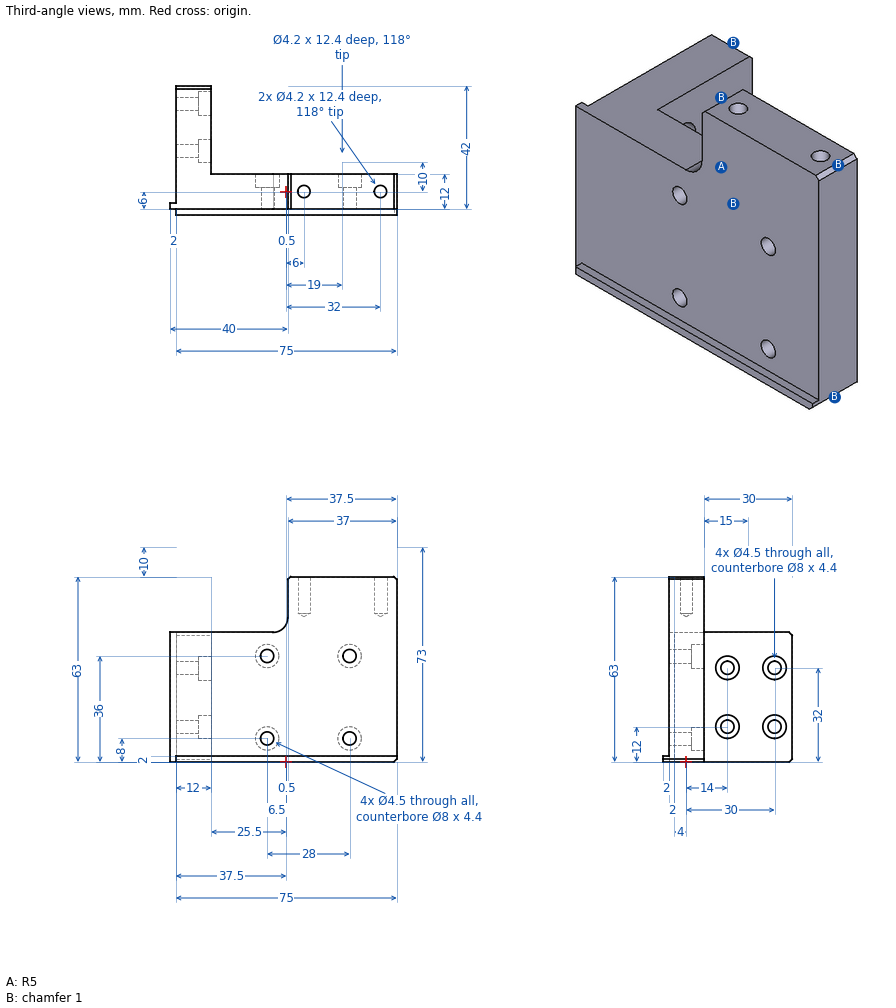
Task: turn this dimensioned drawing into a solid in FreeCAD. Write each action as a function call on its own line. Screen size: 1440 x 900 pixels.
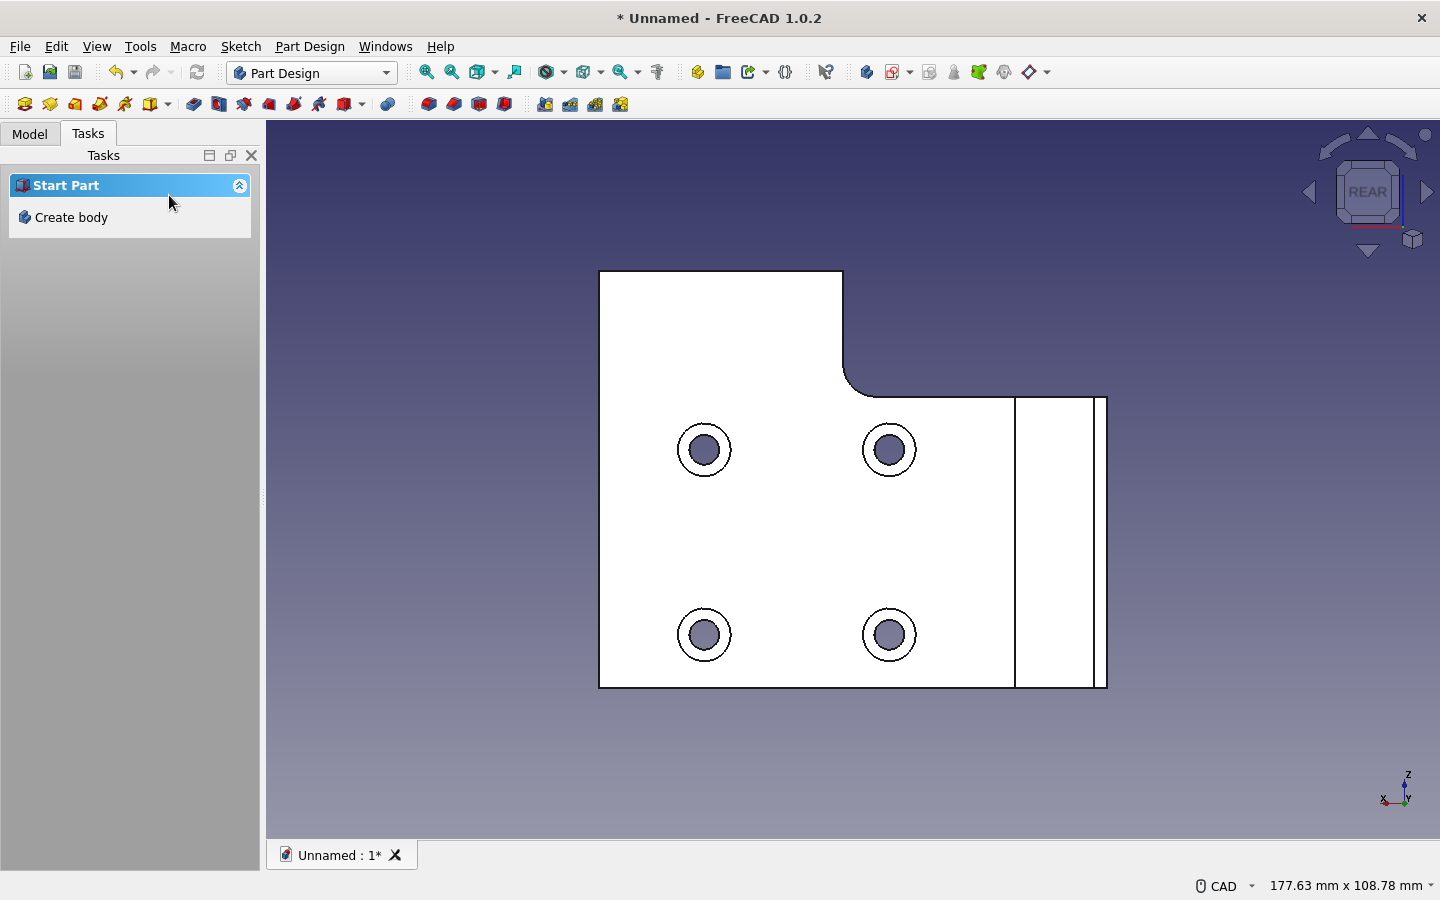
click(1055, 687)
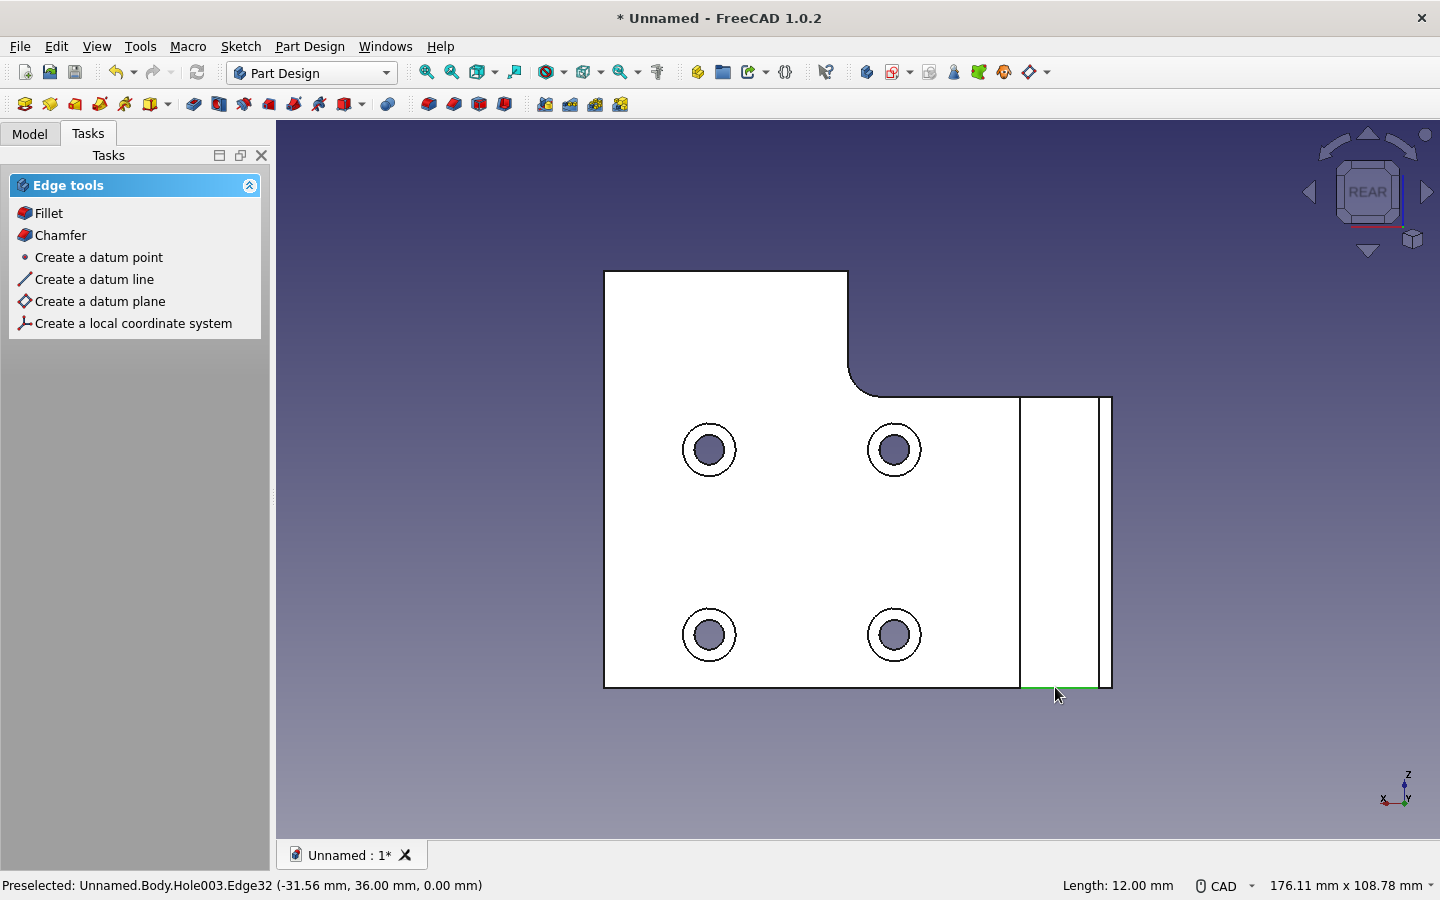
click(1060, 396, ctrl)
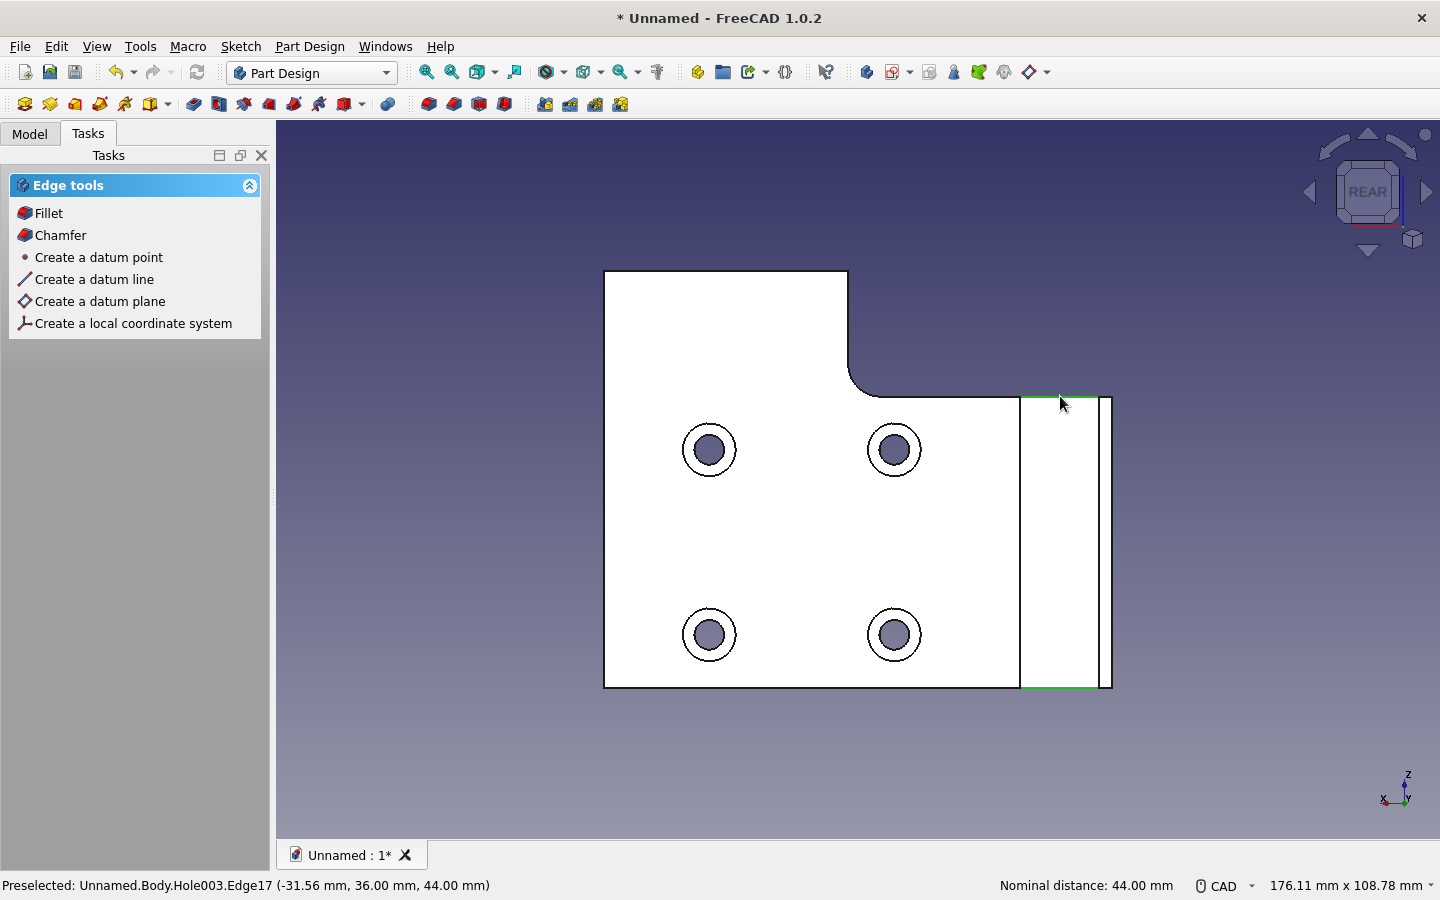
key(0)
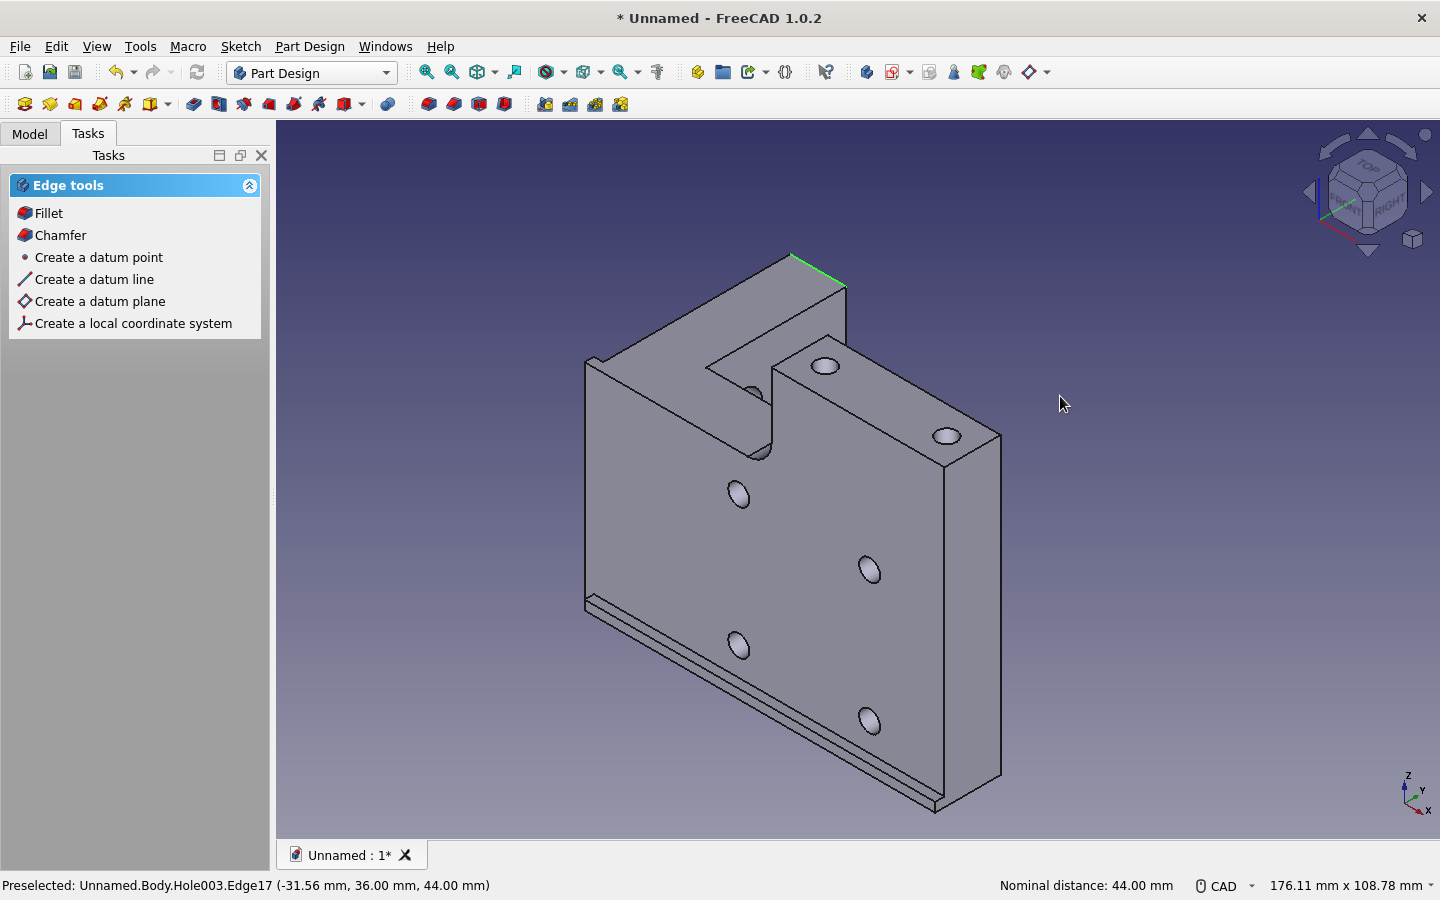
click(973, 450, ctrl)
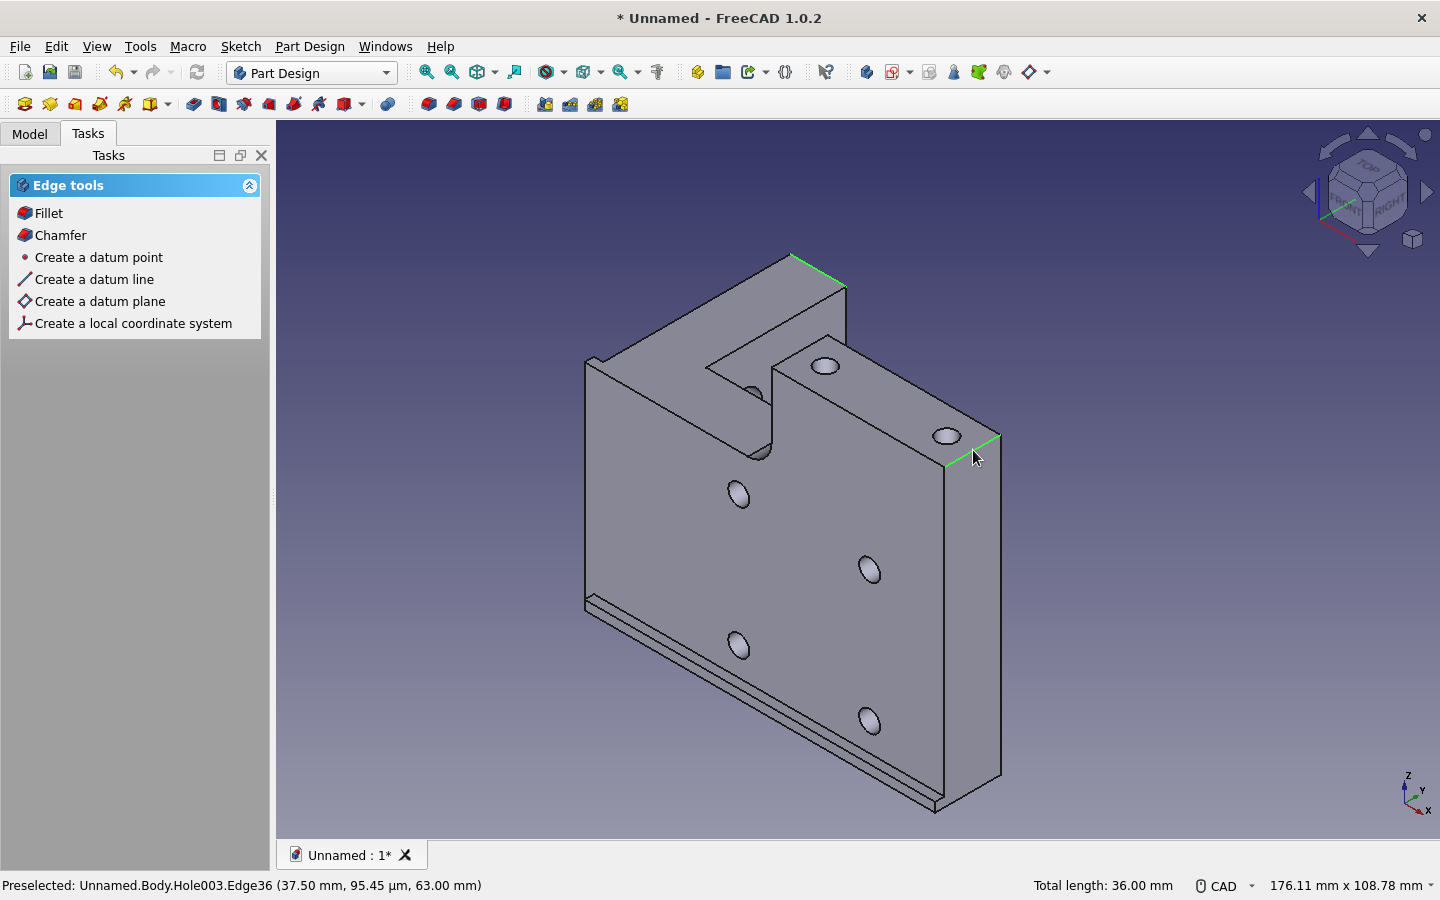
key(2)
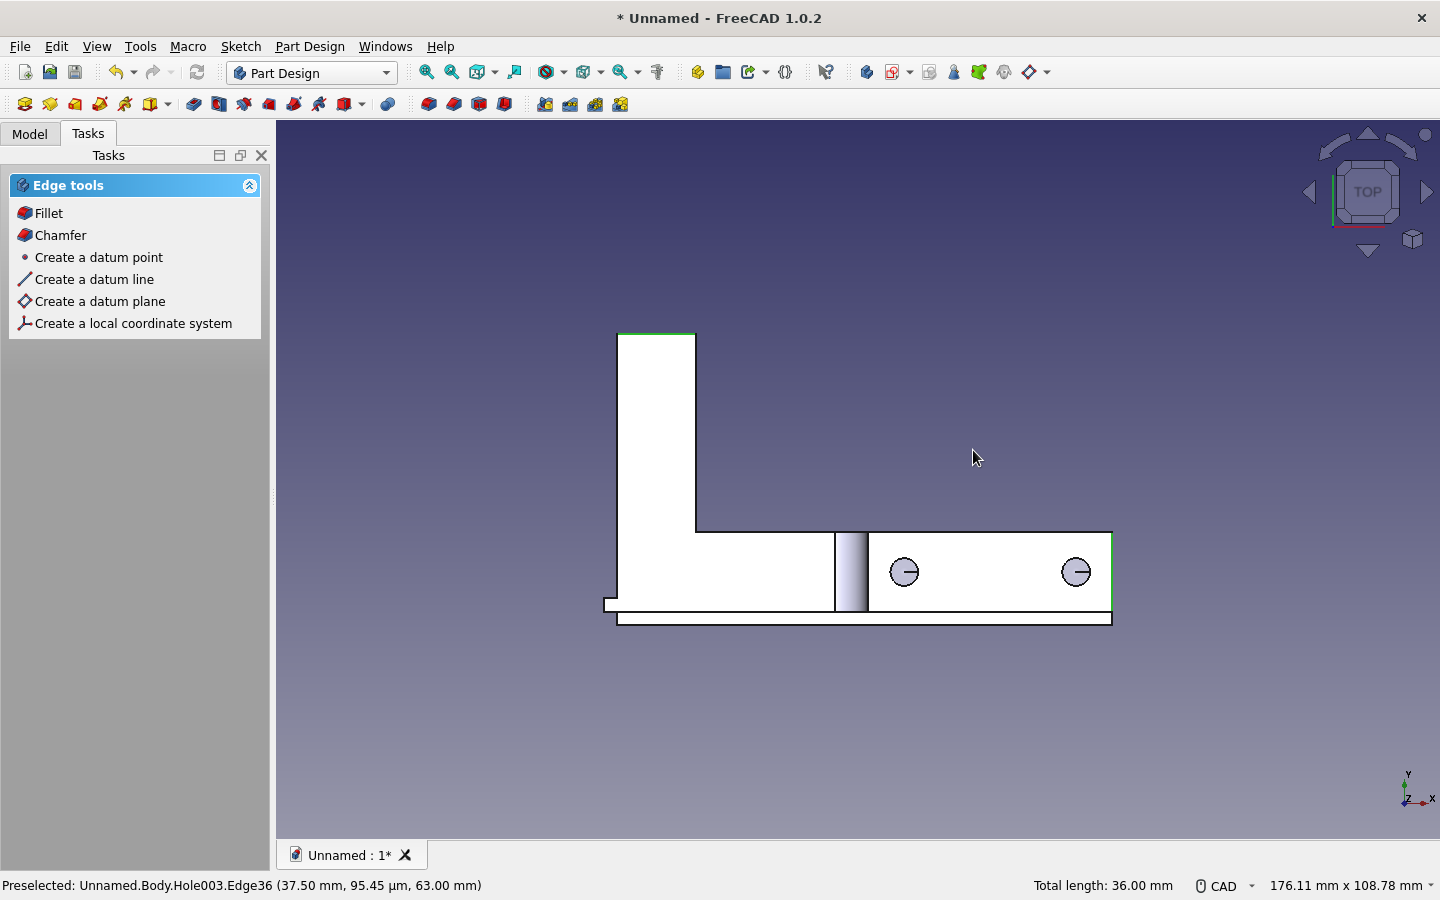
click(427, 72)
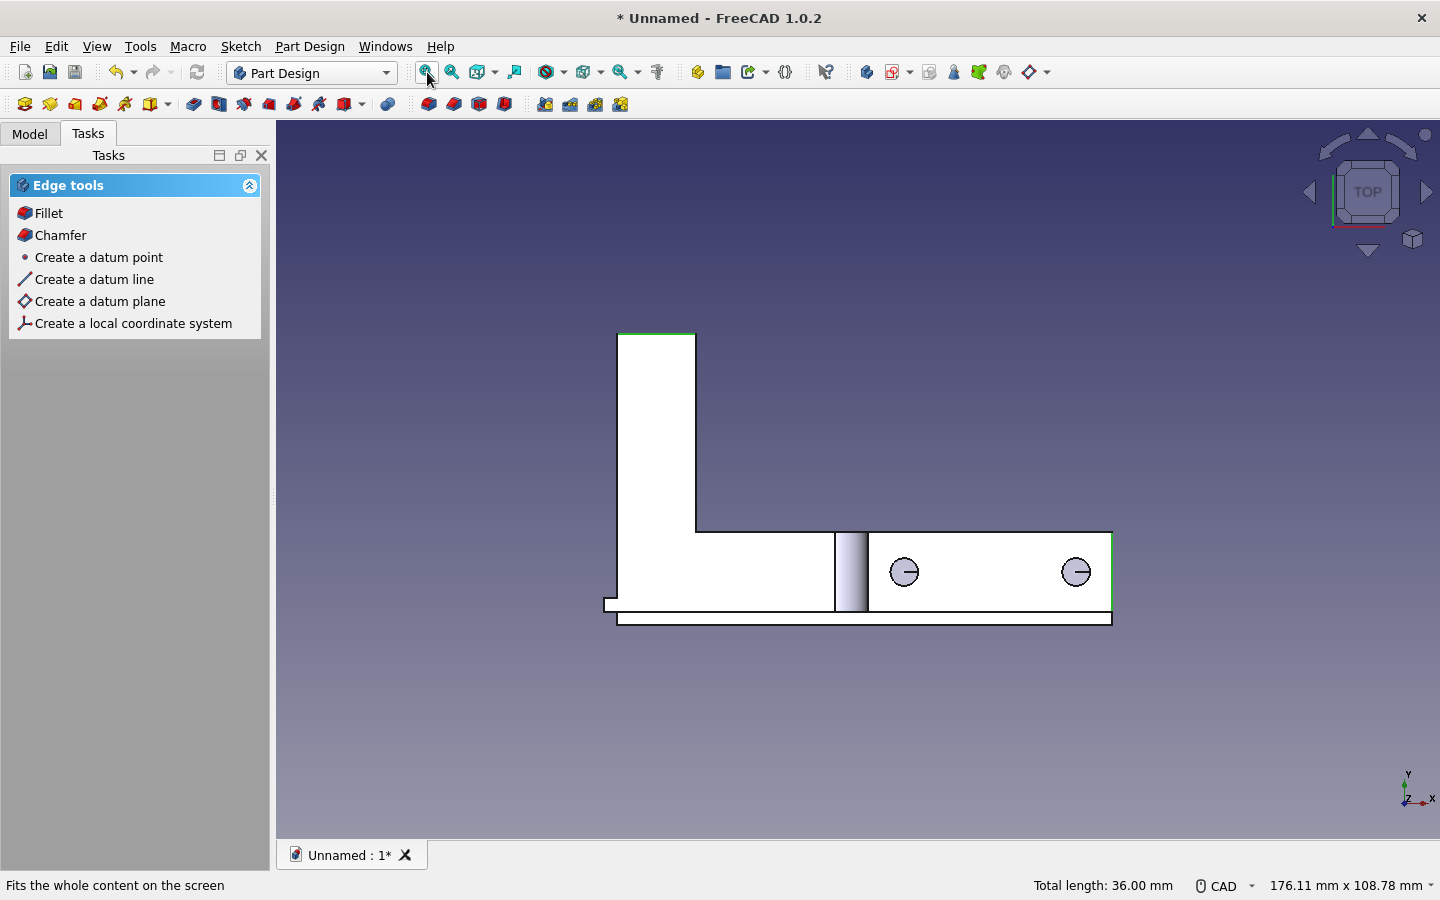
click(868, 571, ctrl)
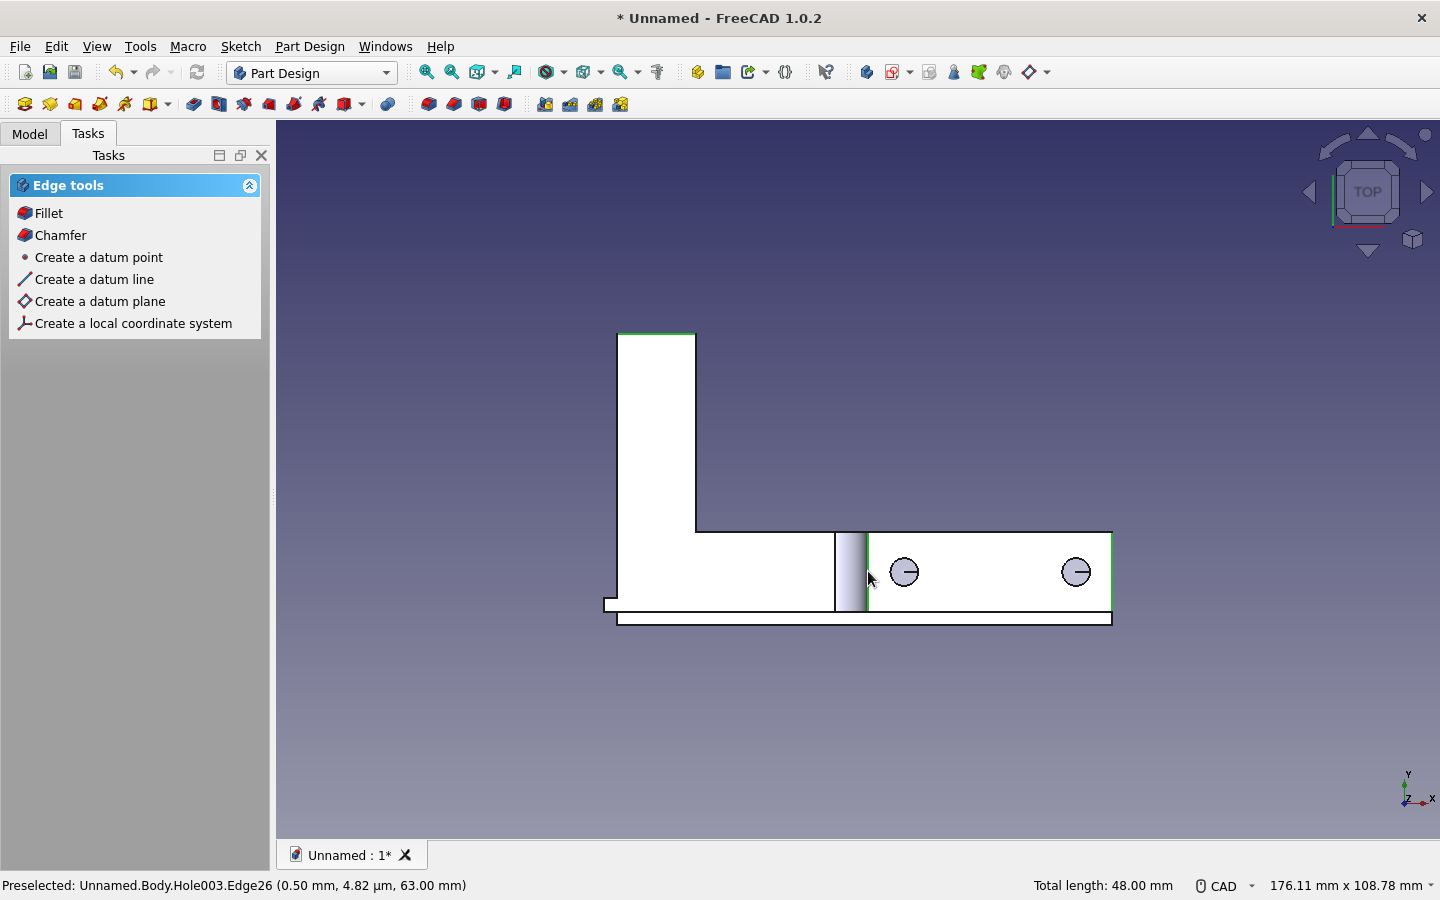
key(1)